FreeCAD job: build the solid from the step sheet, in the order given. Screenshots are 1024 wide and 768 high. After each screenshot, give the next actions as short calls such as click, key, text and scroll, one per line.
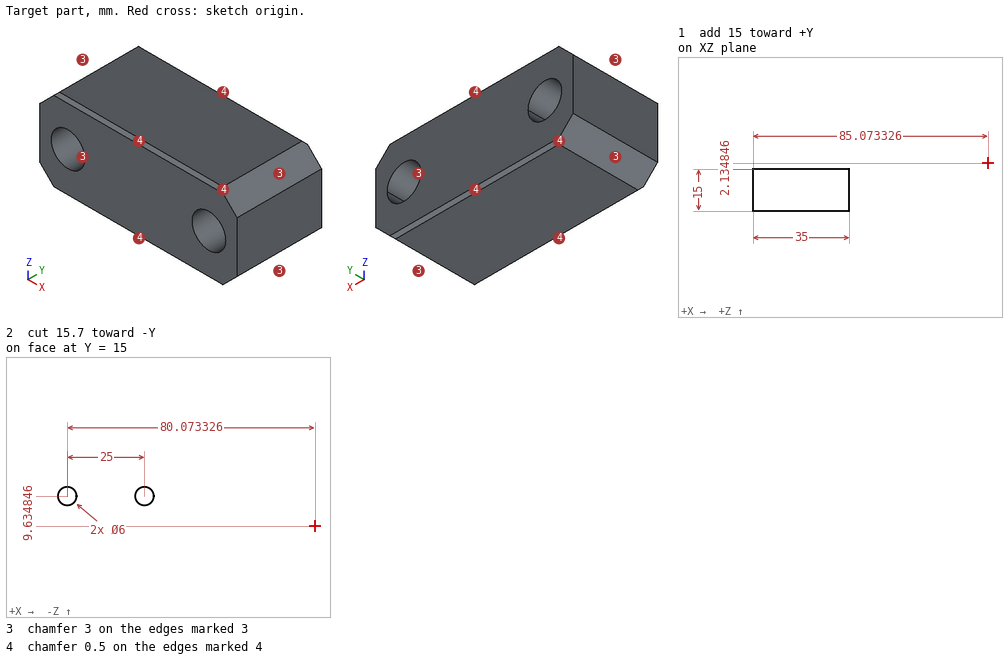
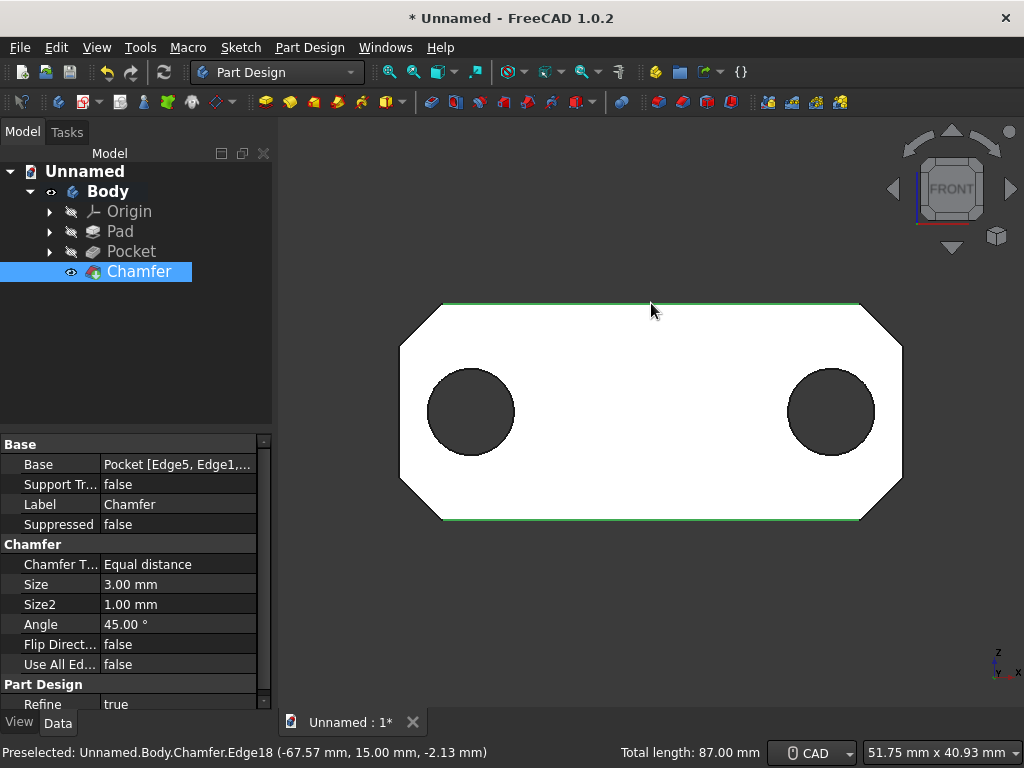
key(3)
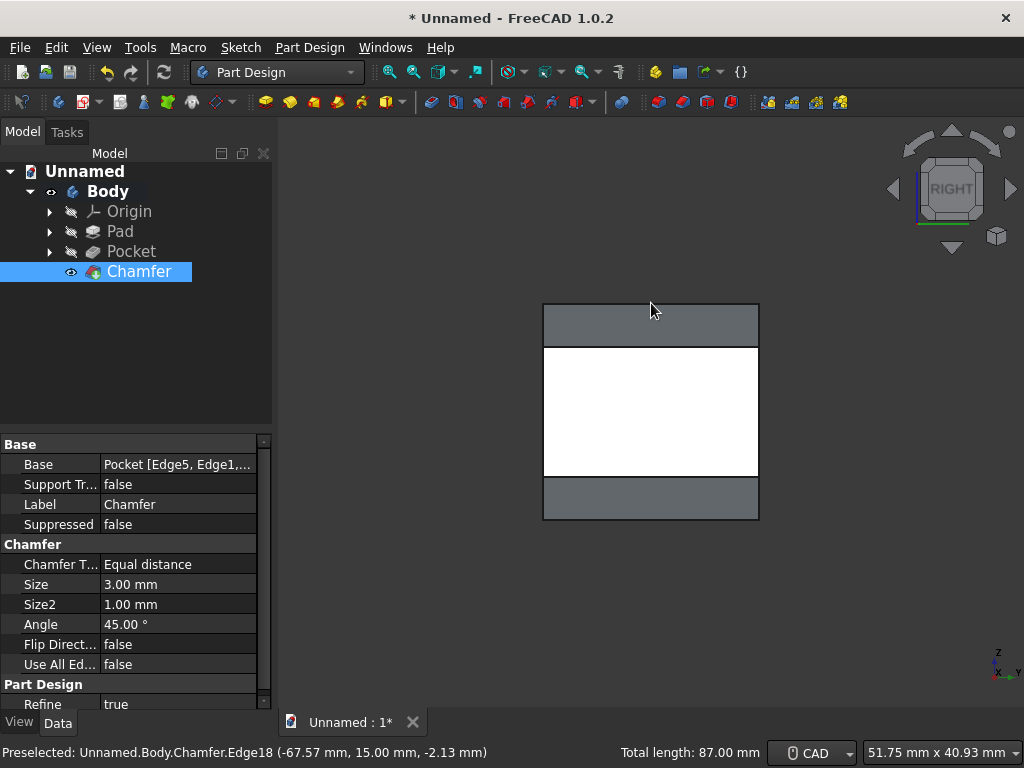
click(390, 72)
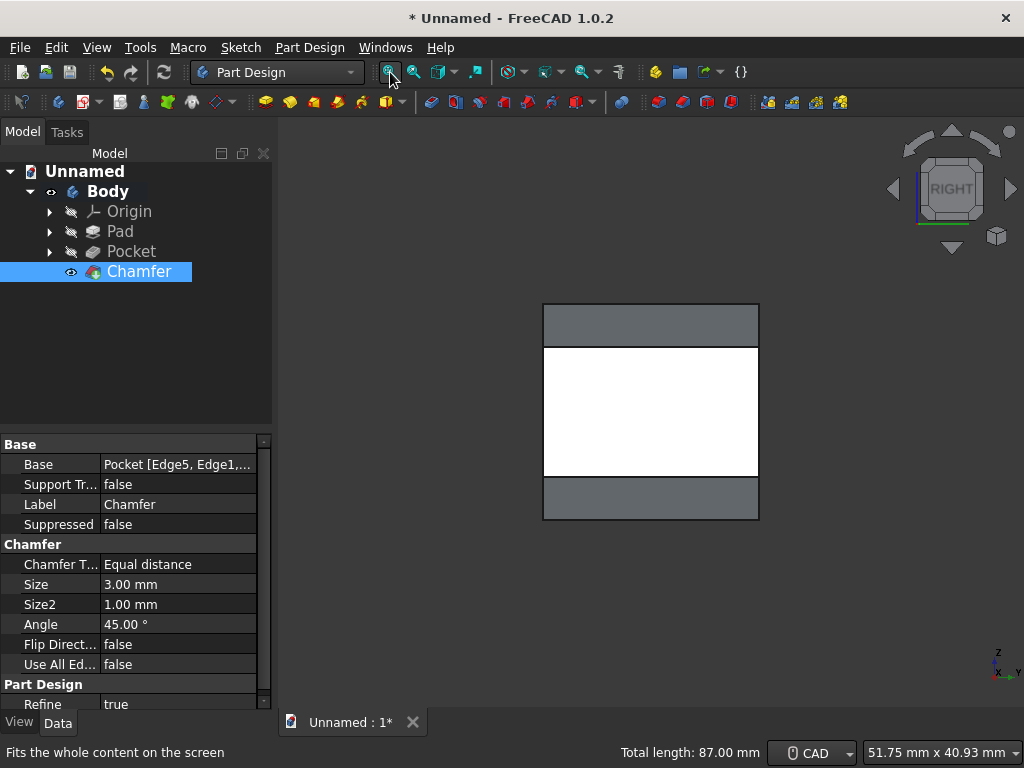
key(5)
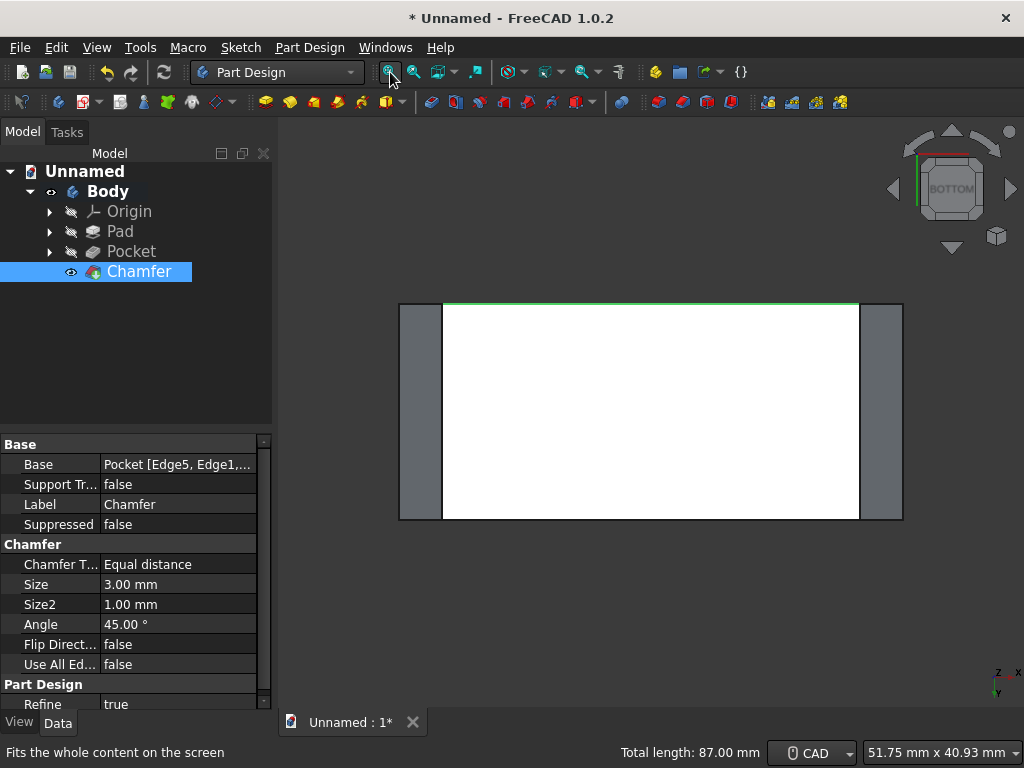
key(4)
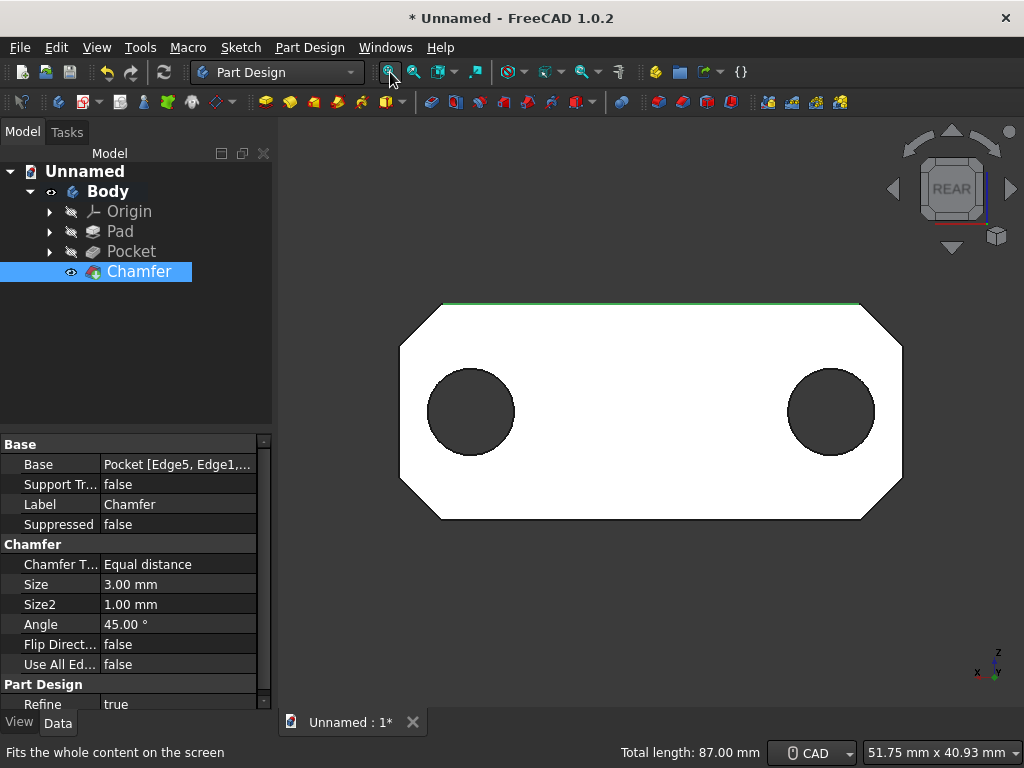
click(651, 519, ctrl)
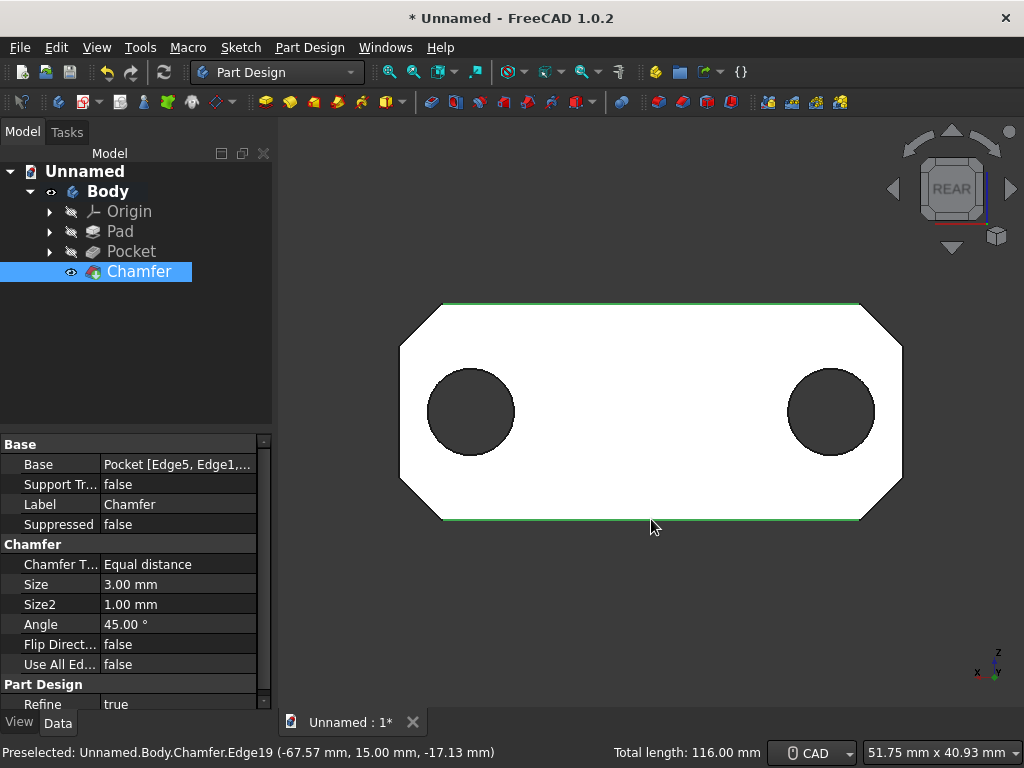
click(684, 102)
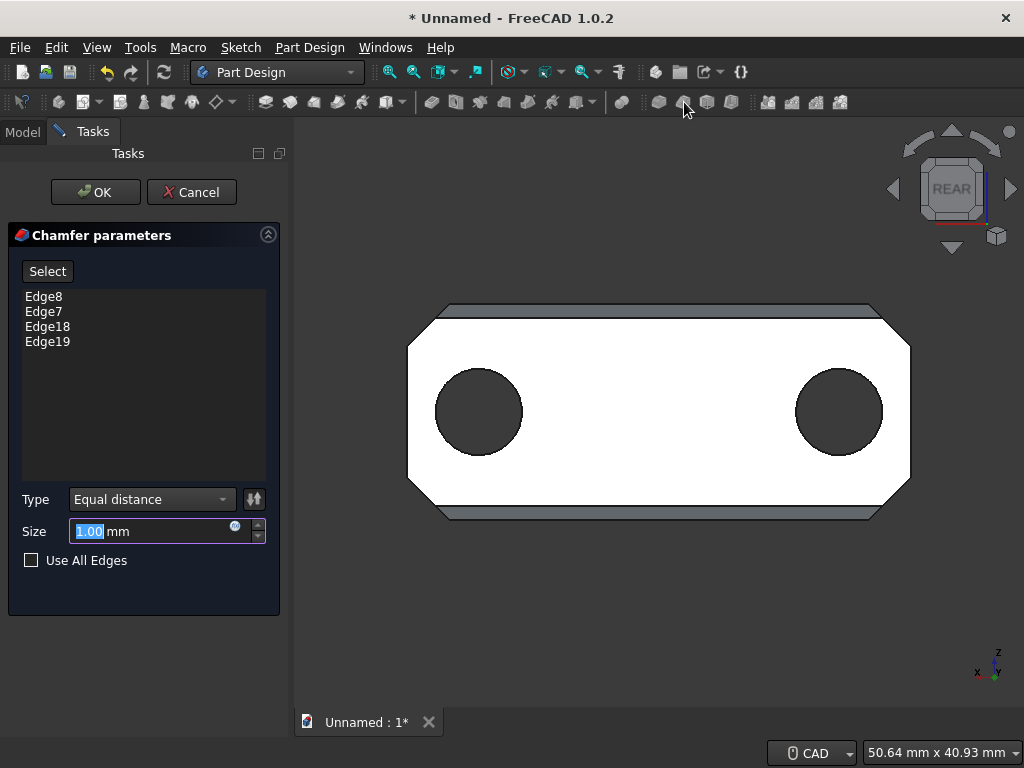
text(0.5)
key(Tab)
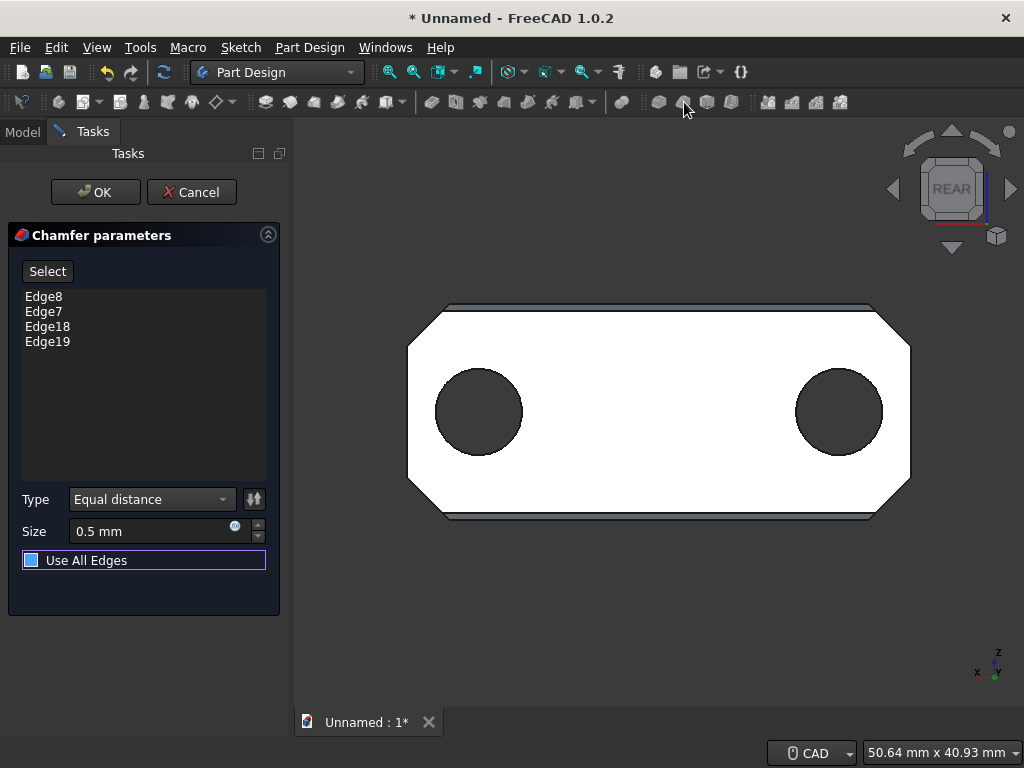
click(96, 192)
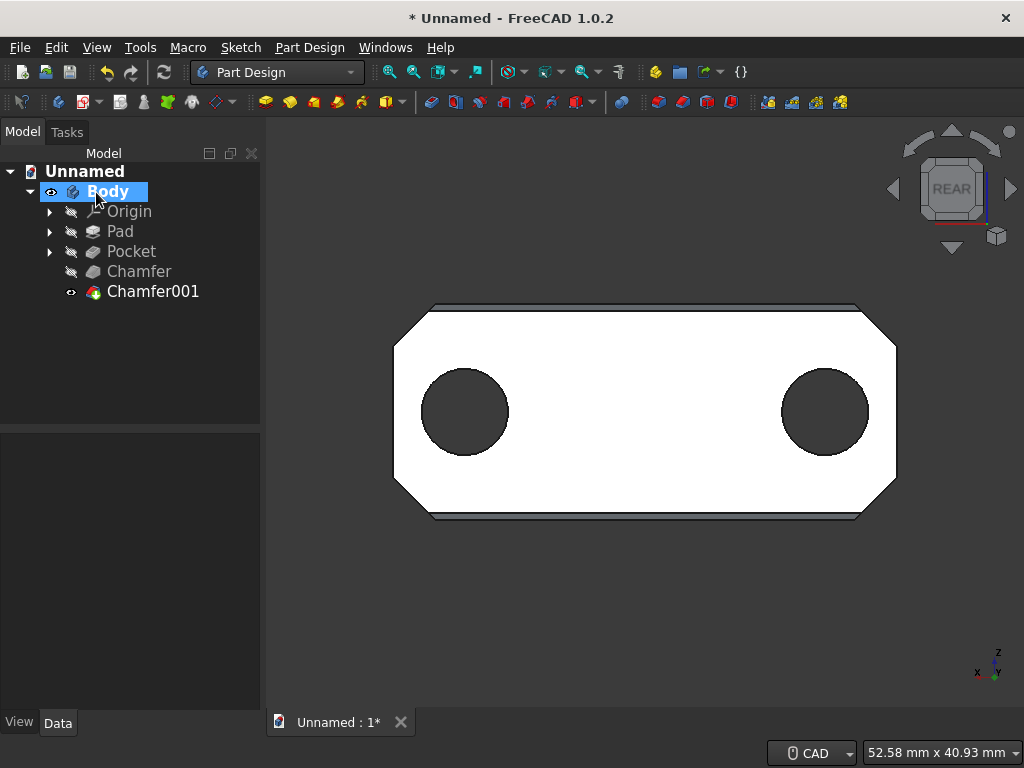
key(0)